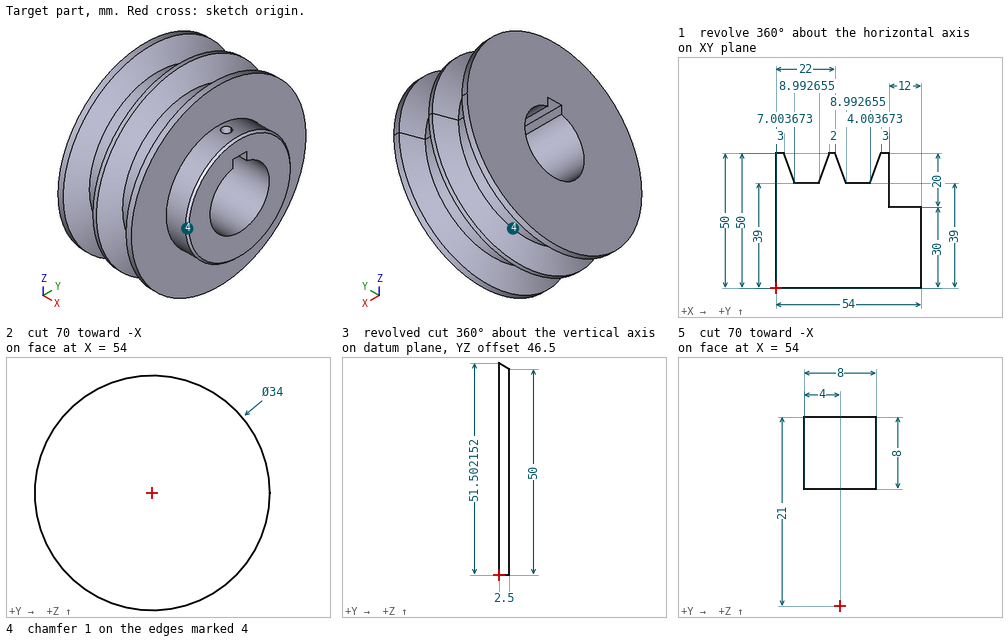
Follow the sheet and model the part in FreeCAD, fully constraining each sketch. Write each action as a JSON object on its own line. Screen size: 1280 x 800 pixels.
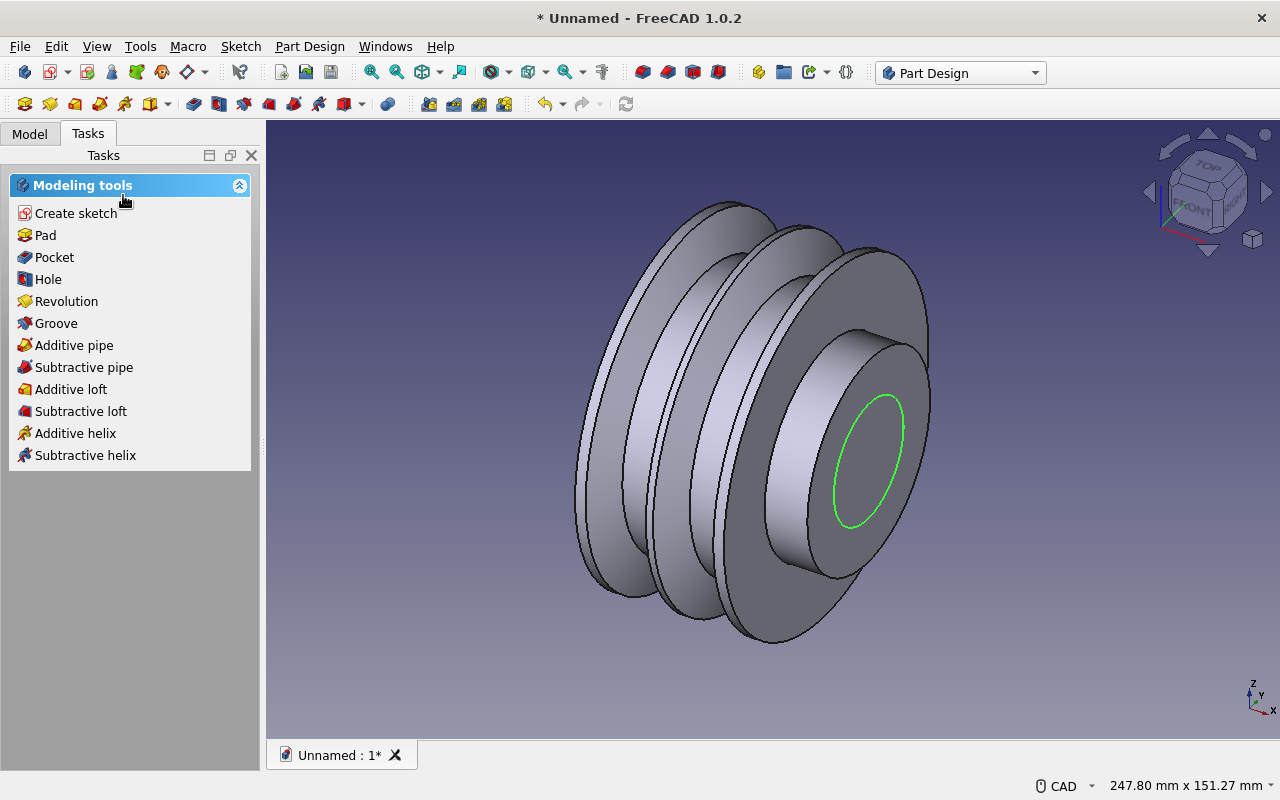
{"action": "left_click", "coordinate": [194, 104]}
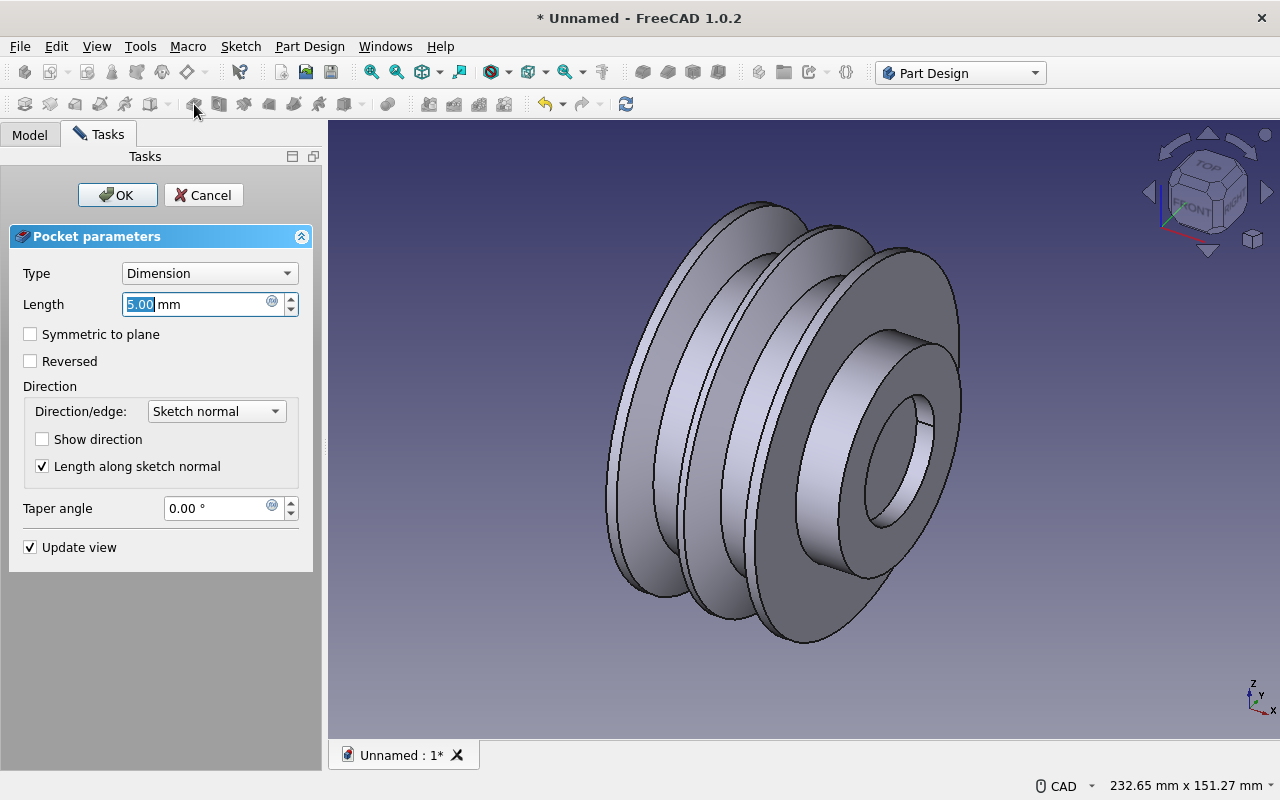
{"action": "type", "text": "70"}
{"action": "key", "text": "Tab"}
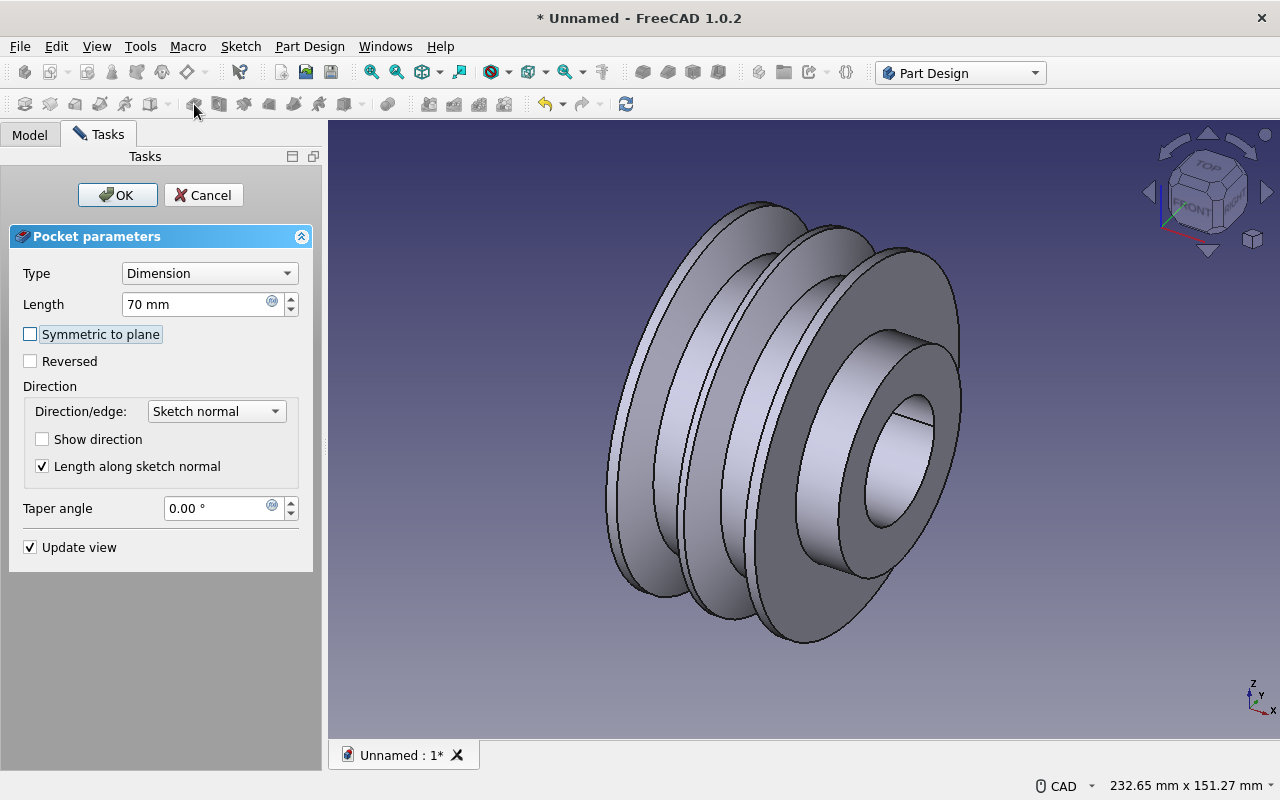
{"action": "left_click", "coordinate": [118, 195]}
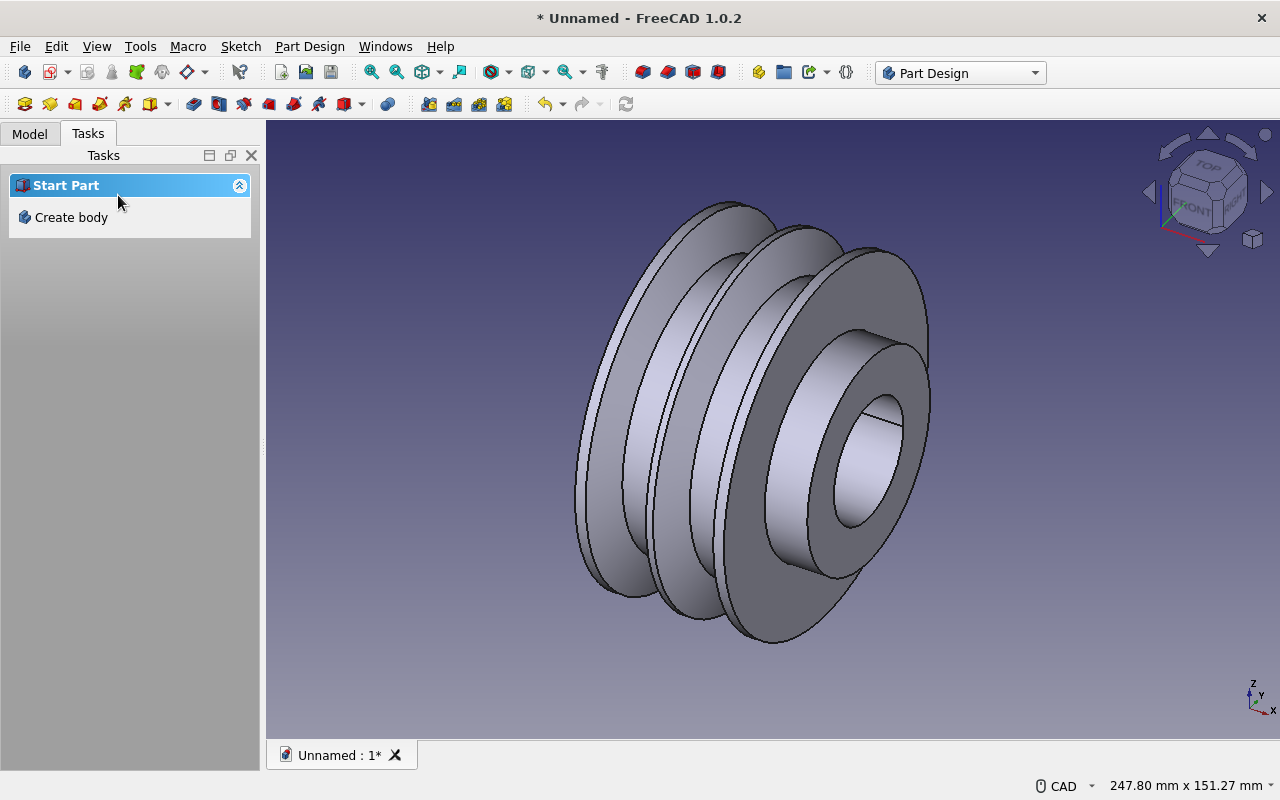
{"action": "left_click", "coordinate": [30, 134]}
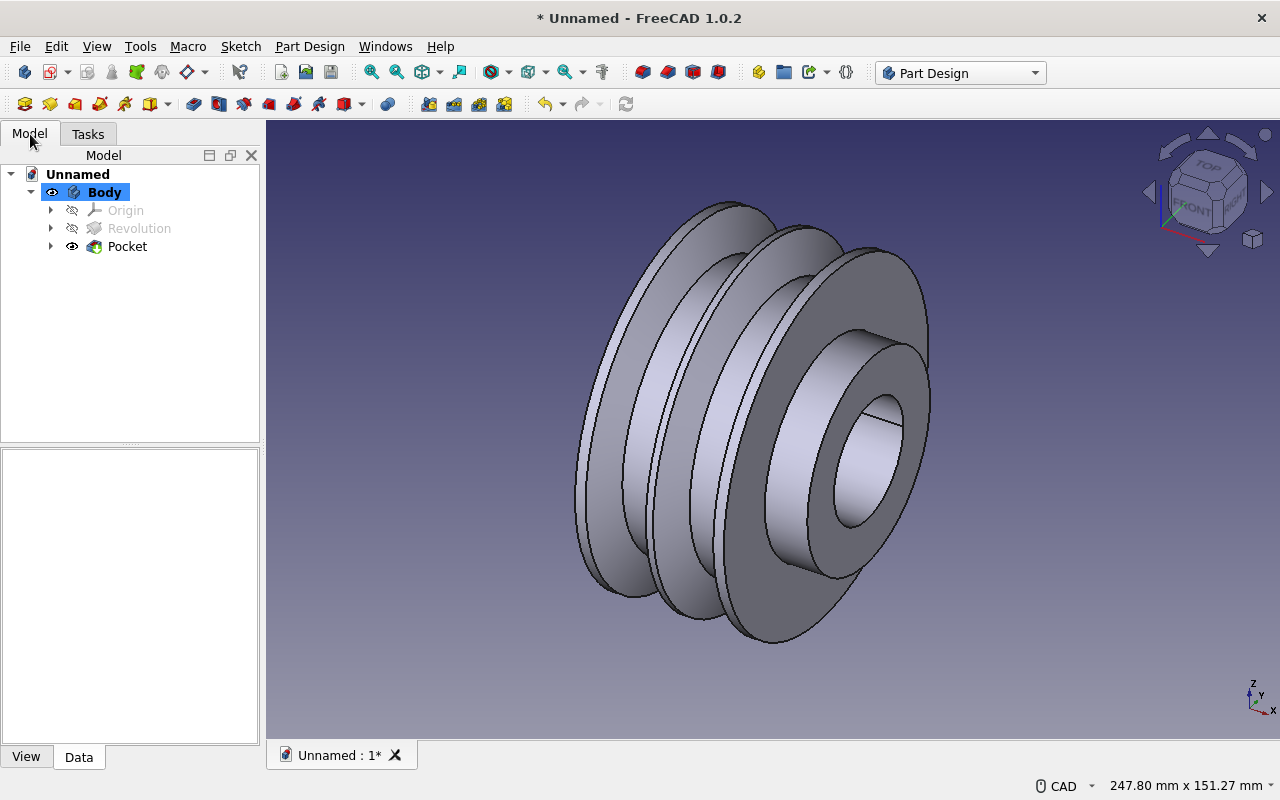
{"action": "left_click", "coordinate": [51, 210]}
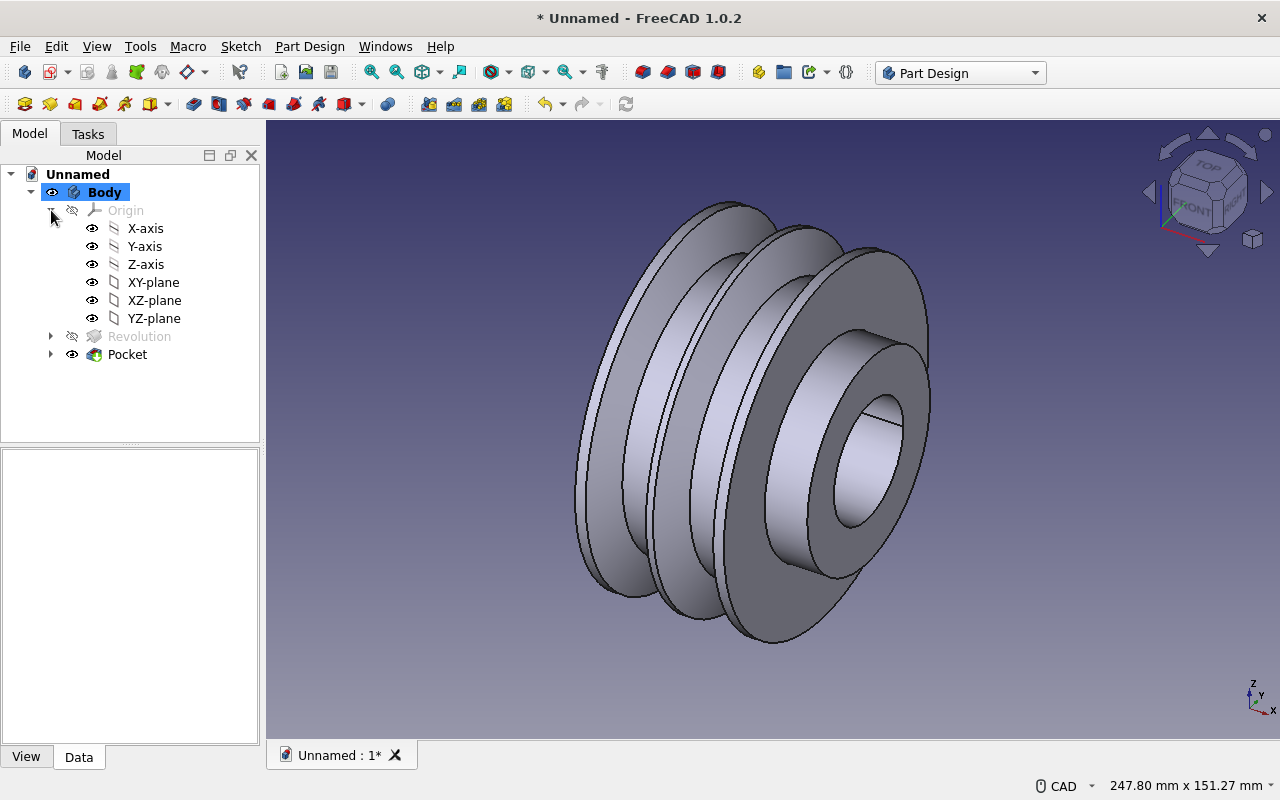
{"action": "left_click", "coordinate": [137, 318]}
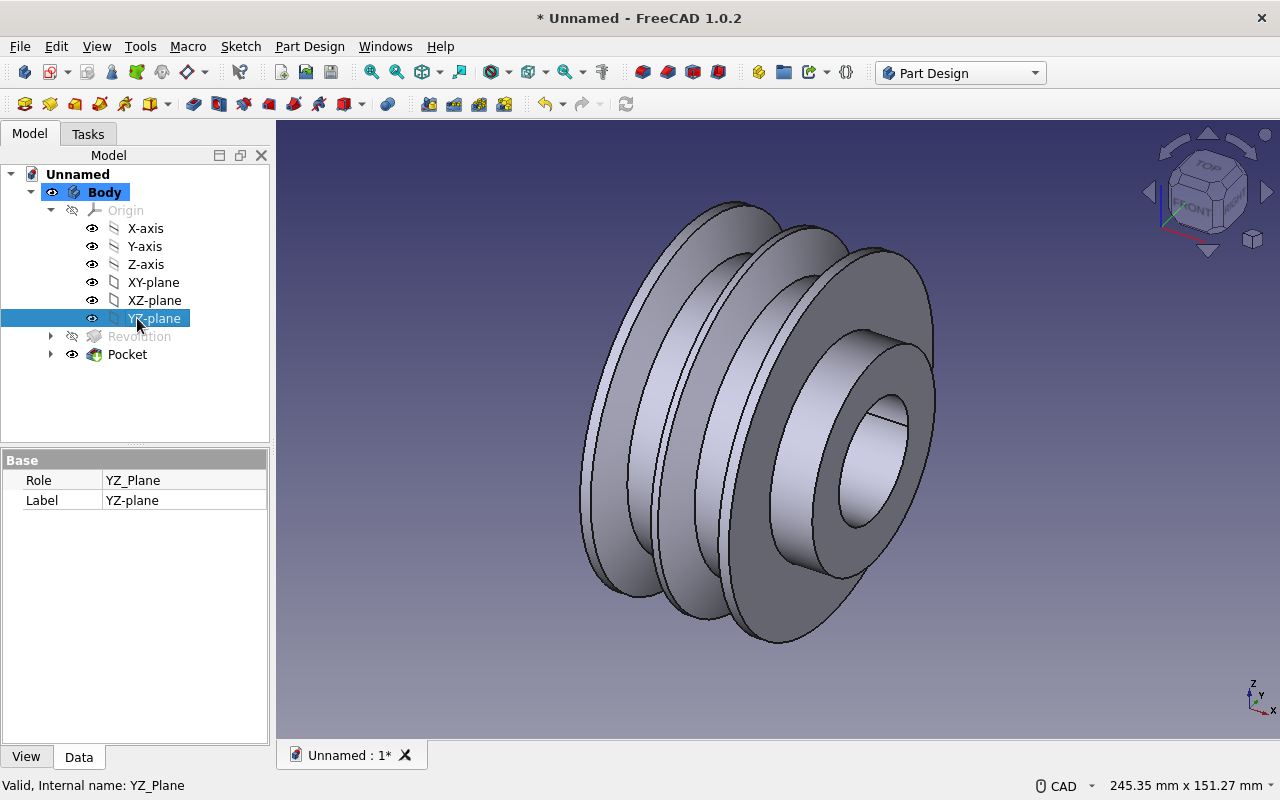
{"action": "left_click", "coordinate": [186, 72]}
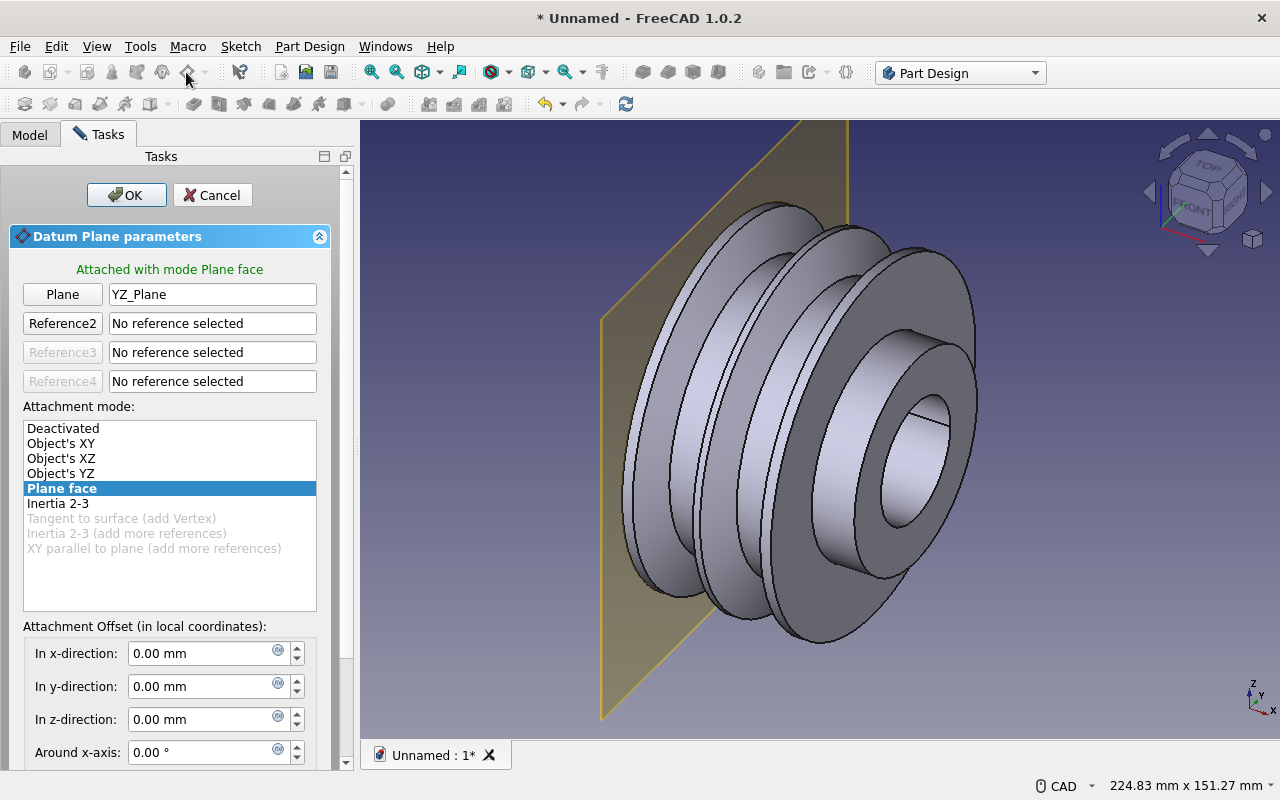
{"action": "triple_click", "coordinate": [210, 720]}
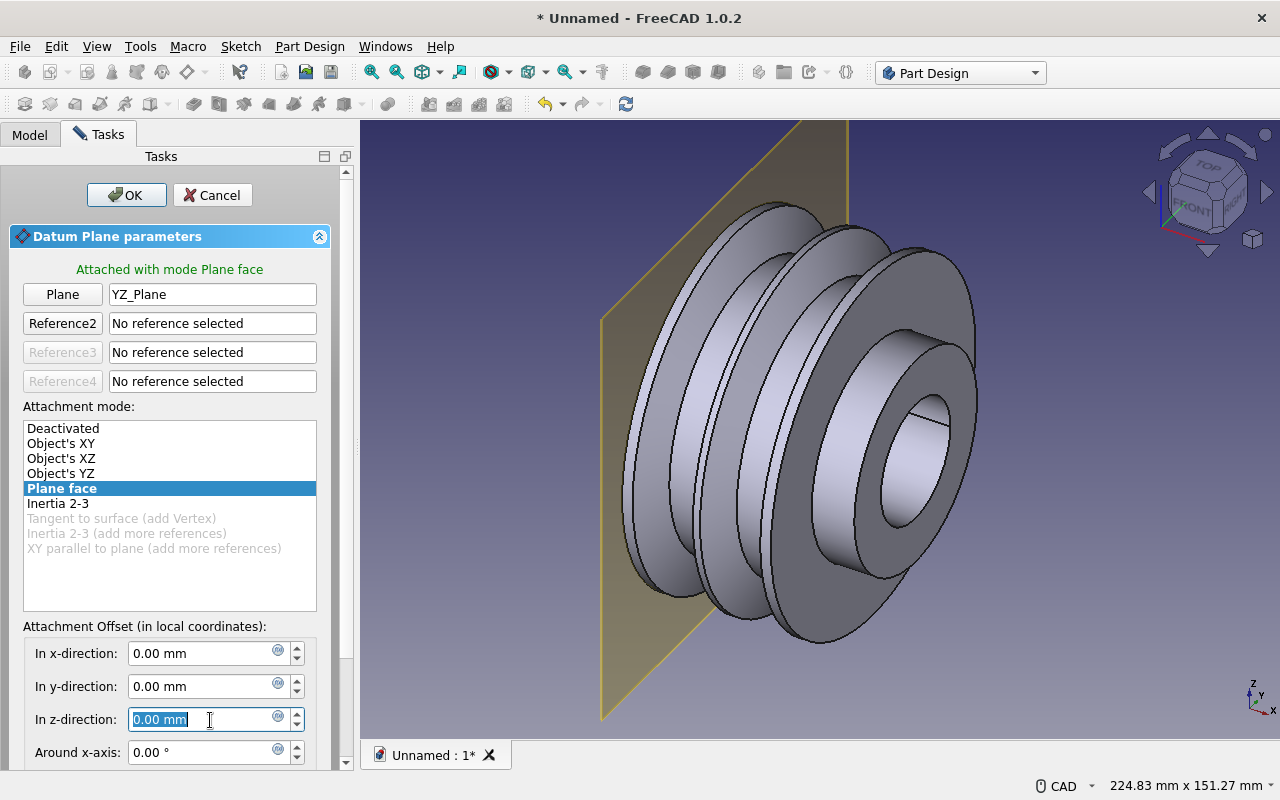
{"action": "type", "text": "46.5"}
{"action": "key", "text": "Tab"}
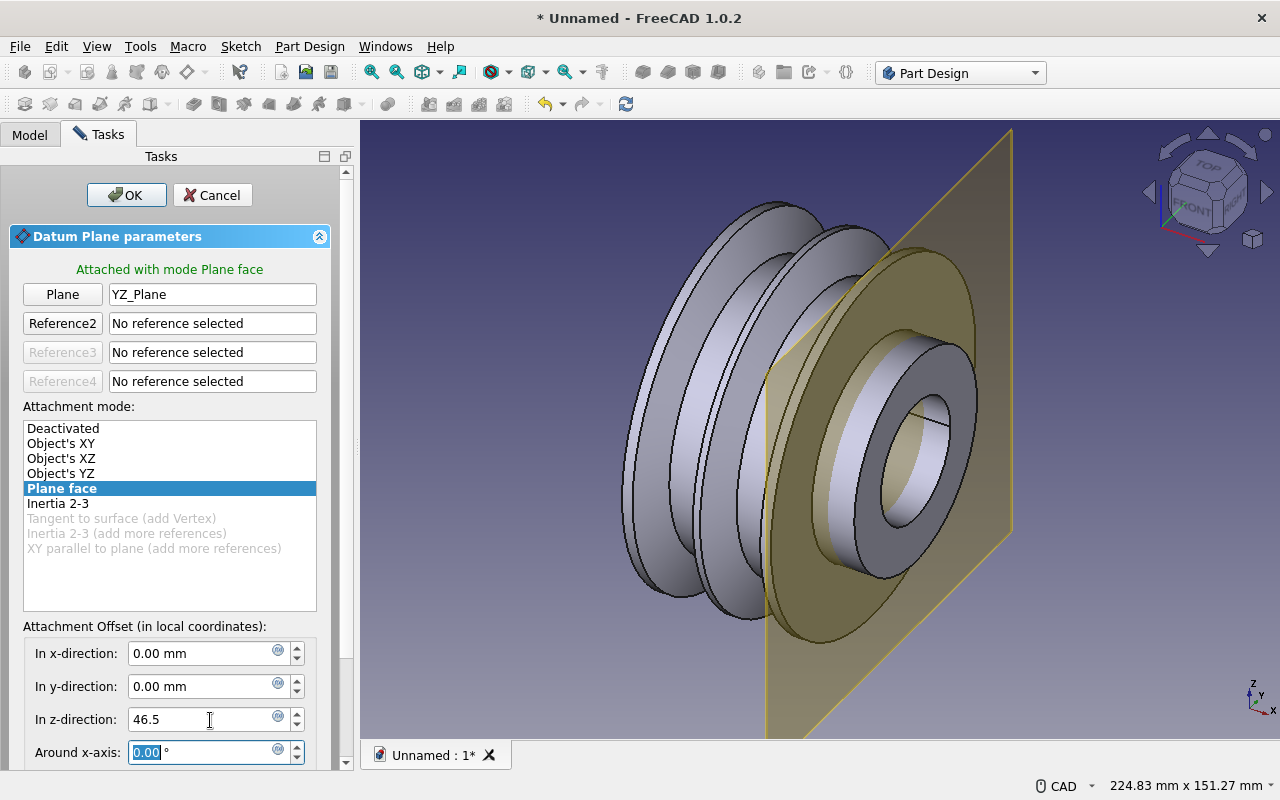
{"action": "left_click", "coordinate": [127, 195]}